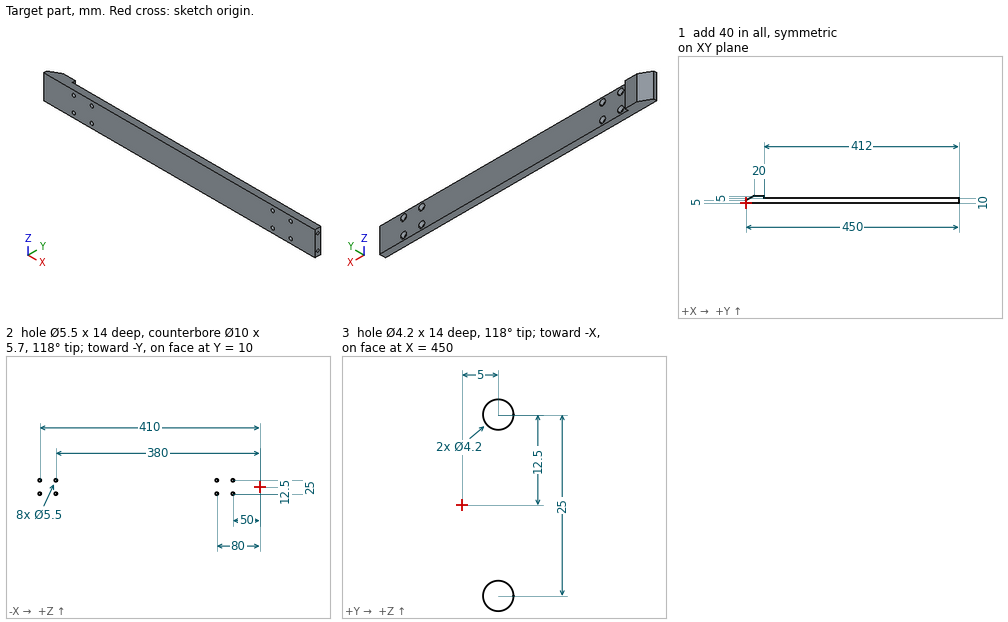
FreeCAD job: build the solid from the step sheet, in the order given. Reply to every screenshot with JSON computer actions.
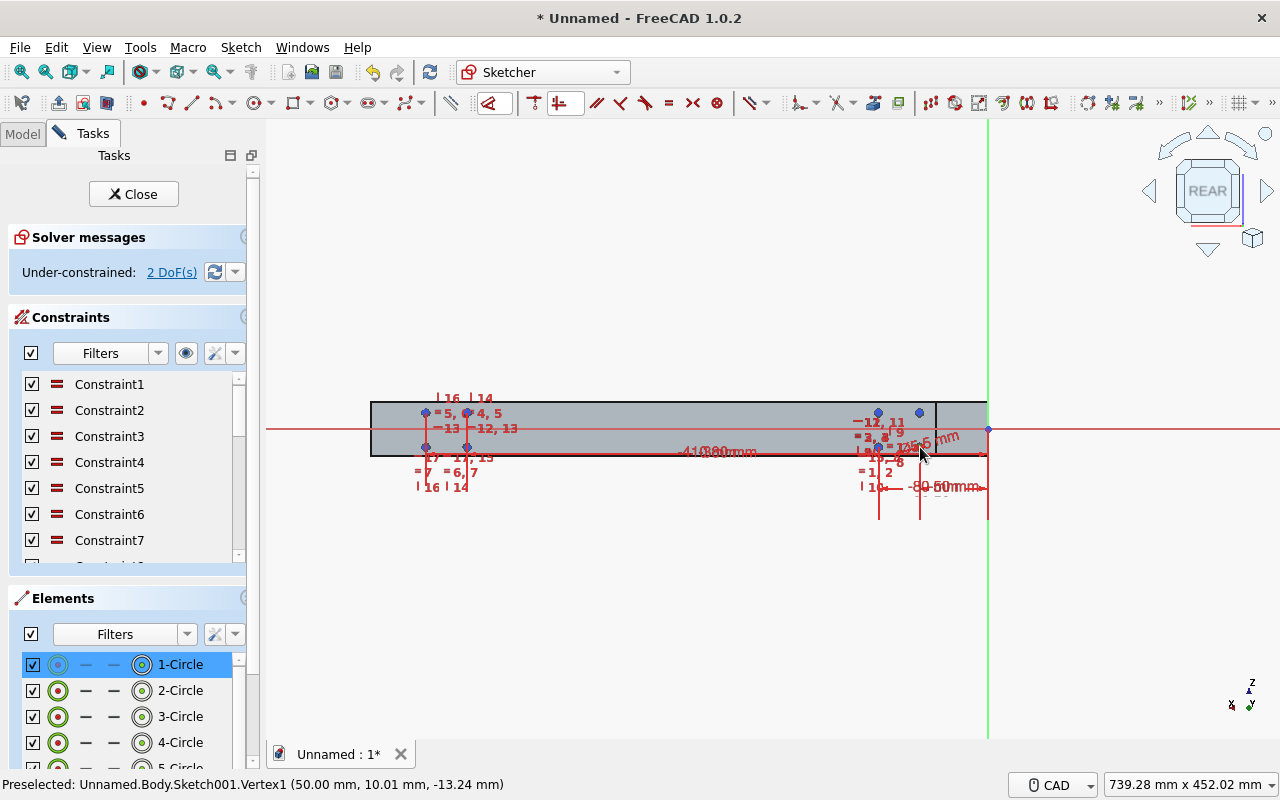
{"action": "left_click", "coordinate": [920, 413]}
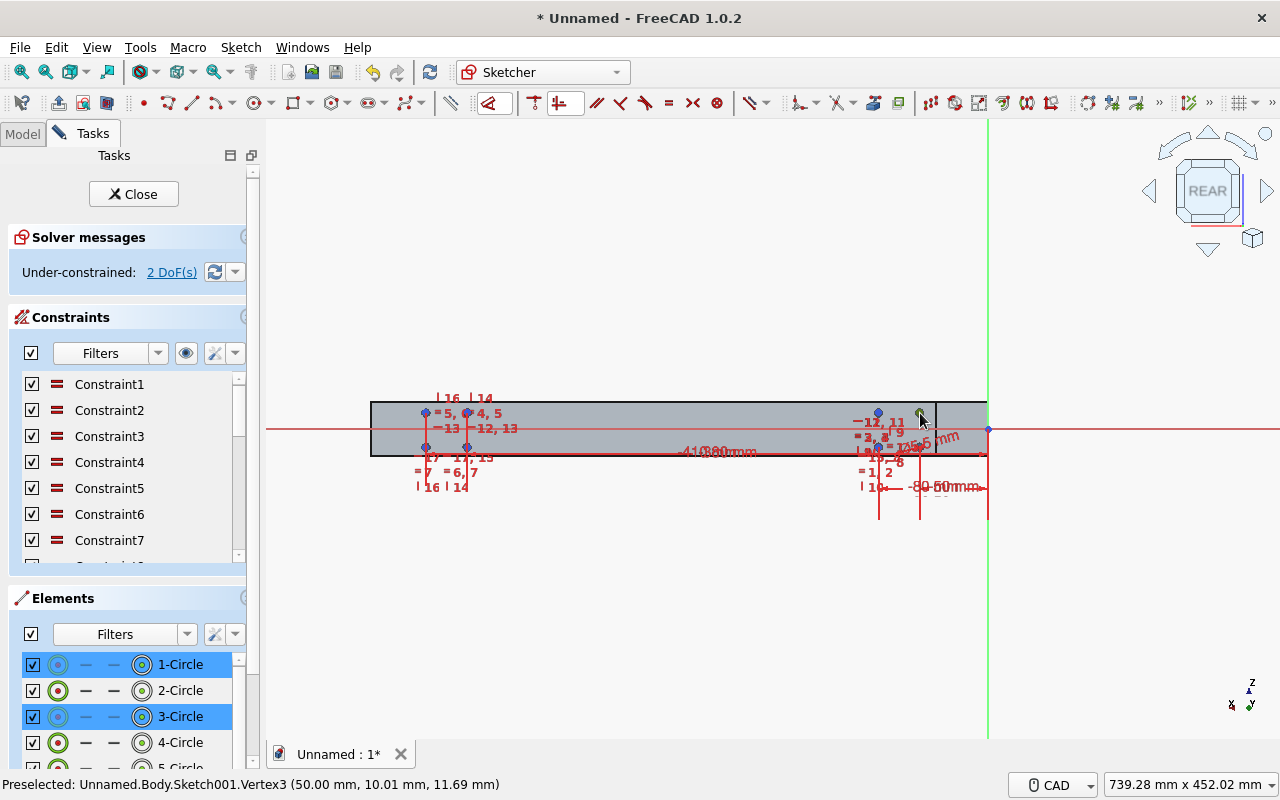
{"action": "key", "text": "i"}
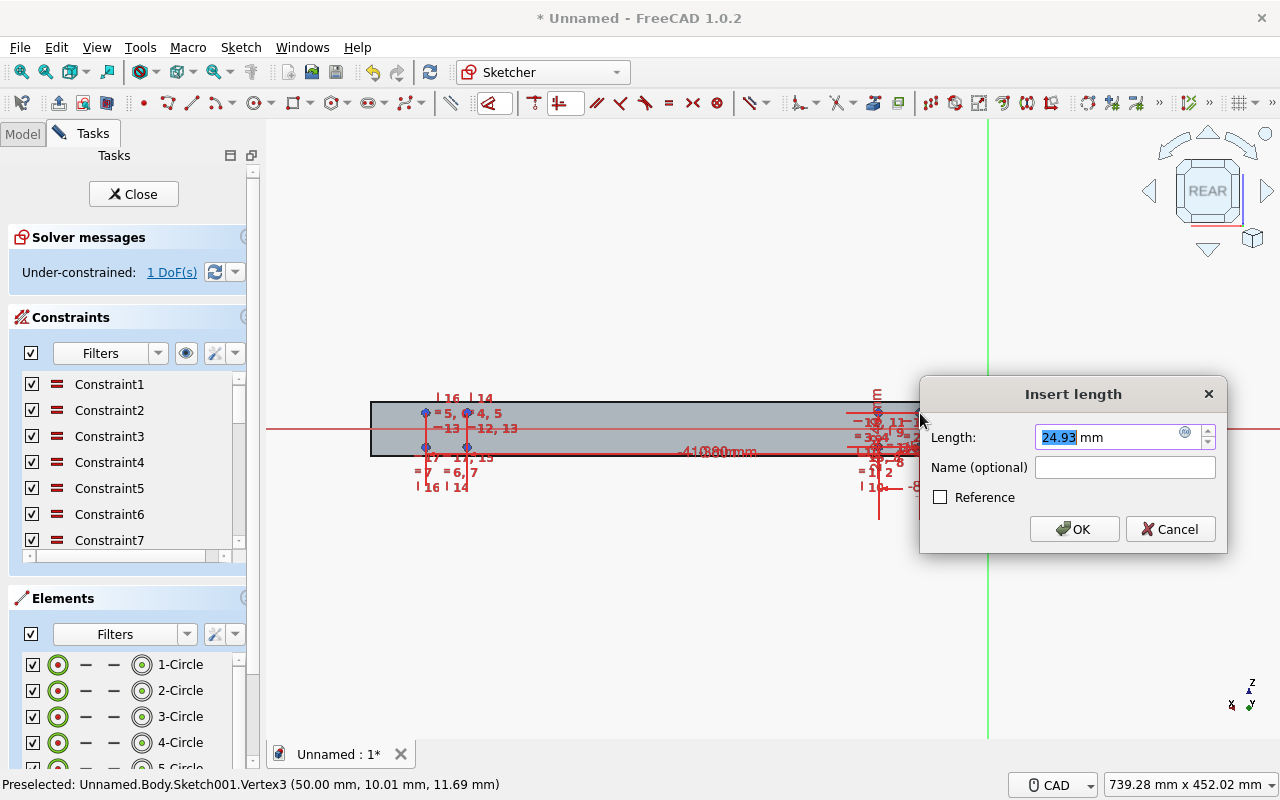
{"action": "type", "text": "25"}
{"action": "key", "text": "Return"}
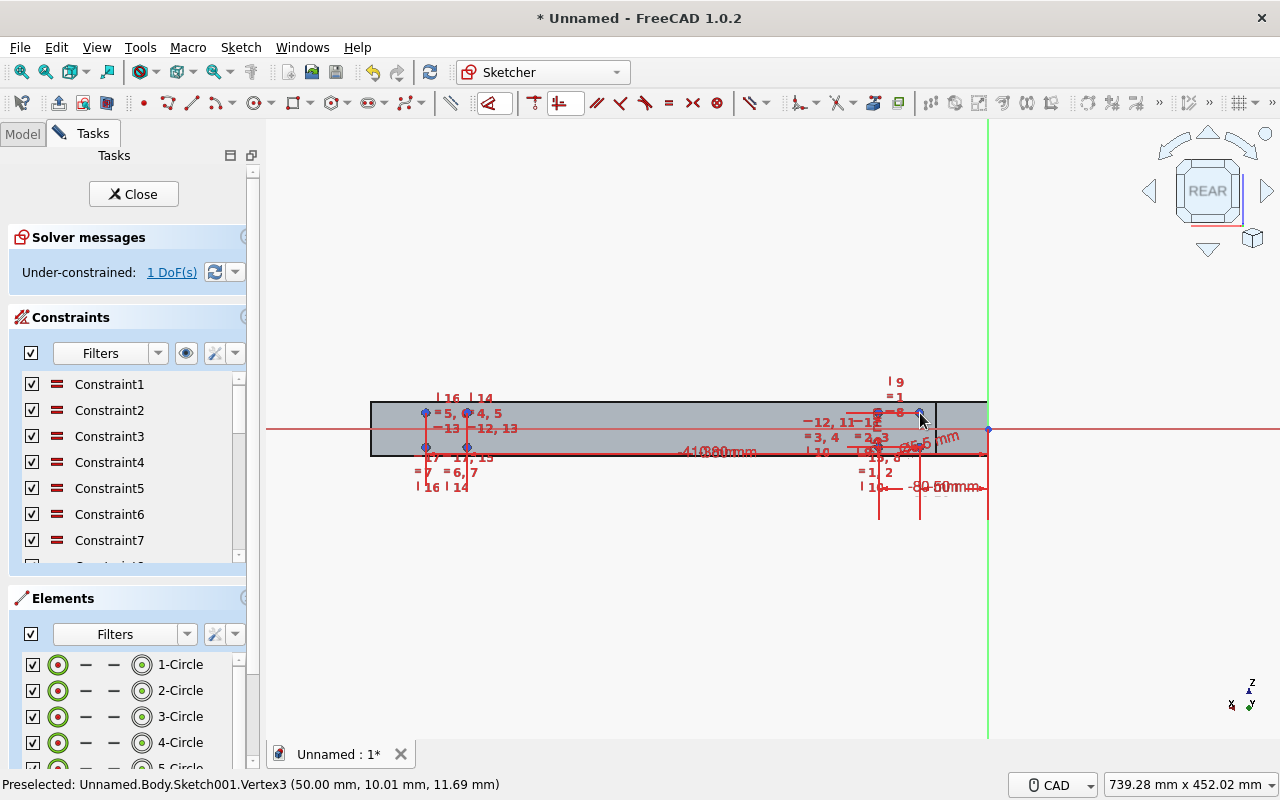
{"action": "scroll", "coordinate": [920, 447], "scroll_direction": "up", "scroll_amount": 5}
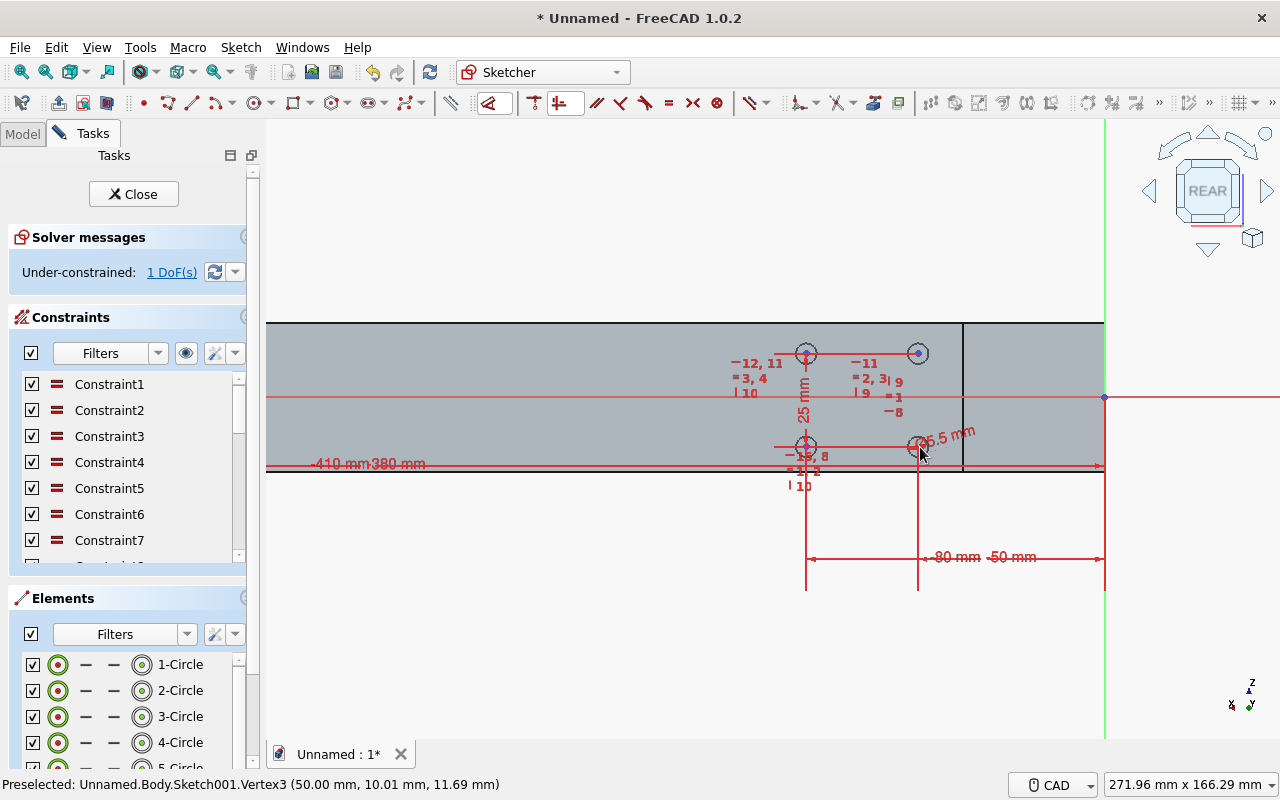
{"action": "left_click", "coordinate": [918, 447]}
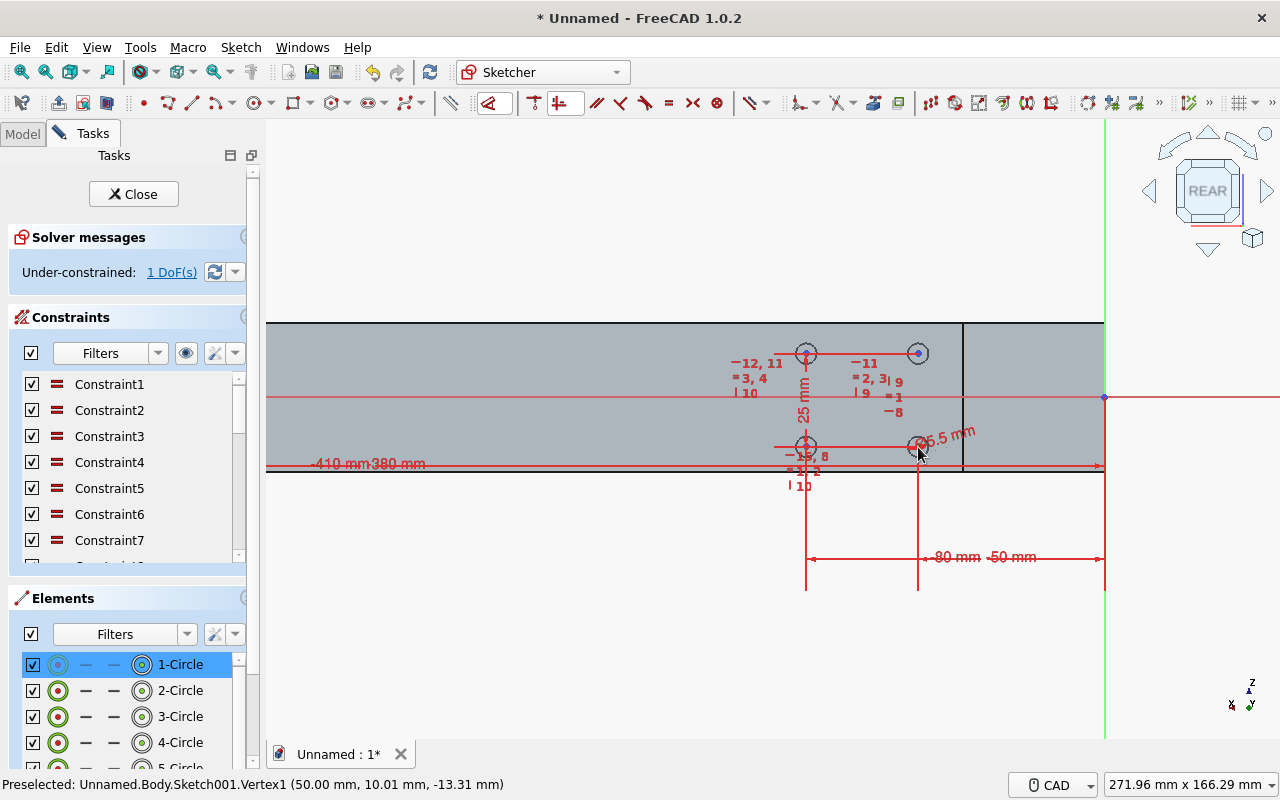
{"action": "key", "text": "i"}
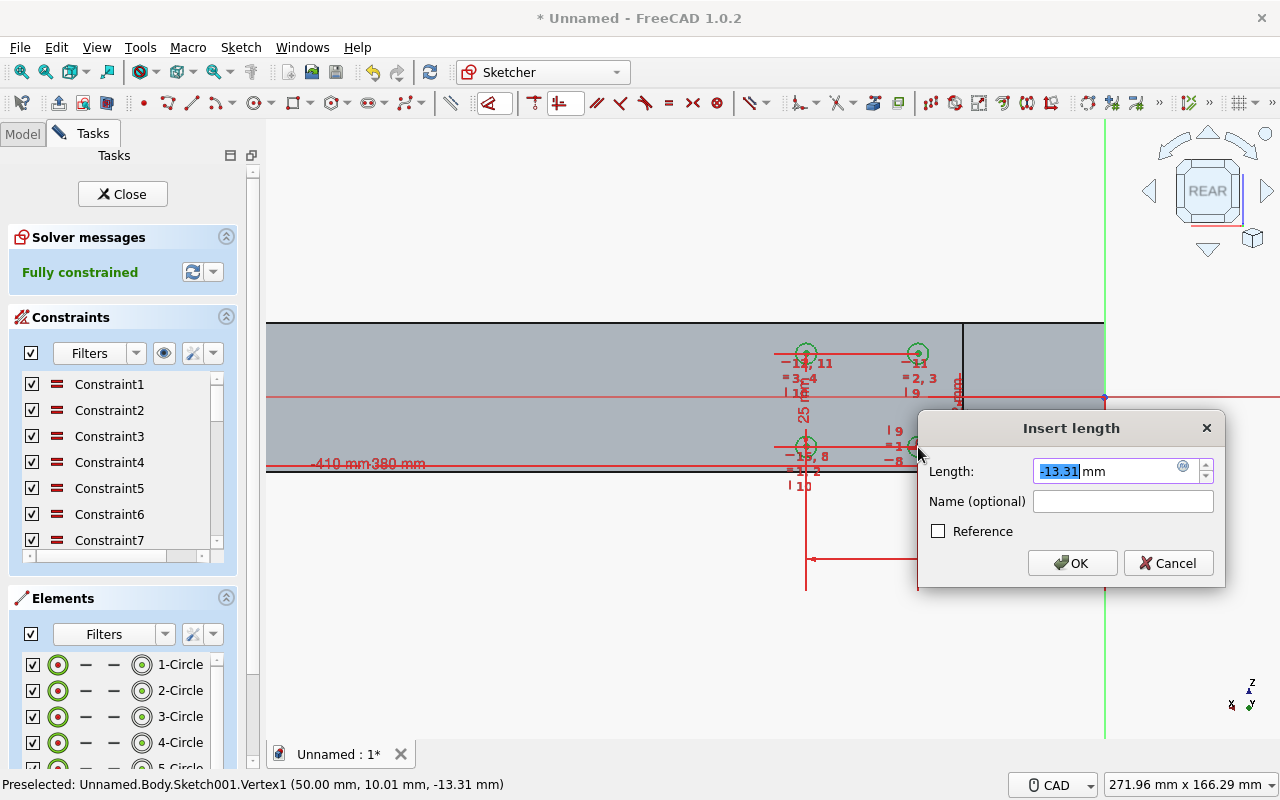
{"action": "type", "text": "-12.5"}
{"action": "key", "text": "Return"}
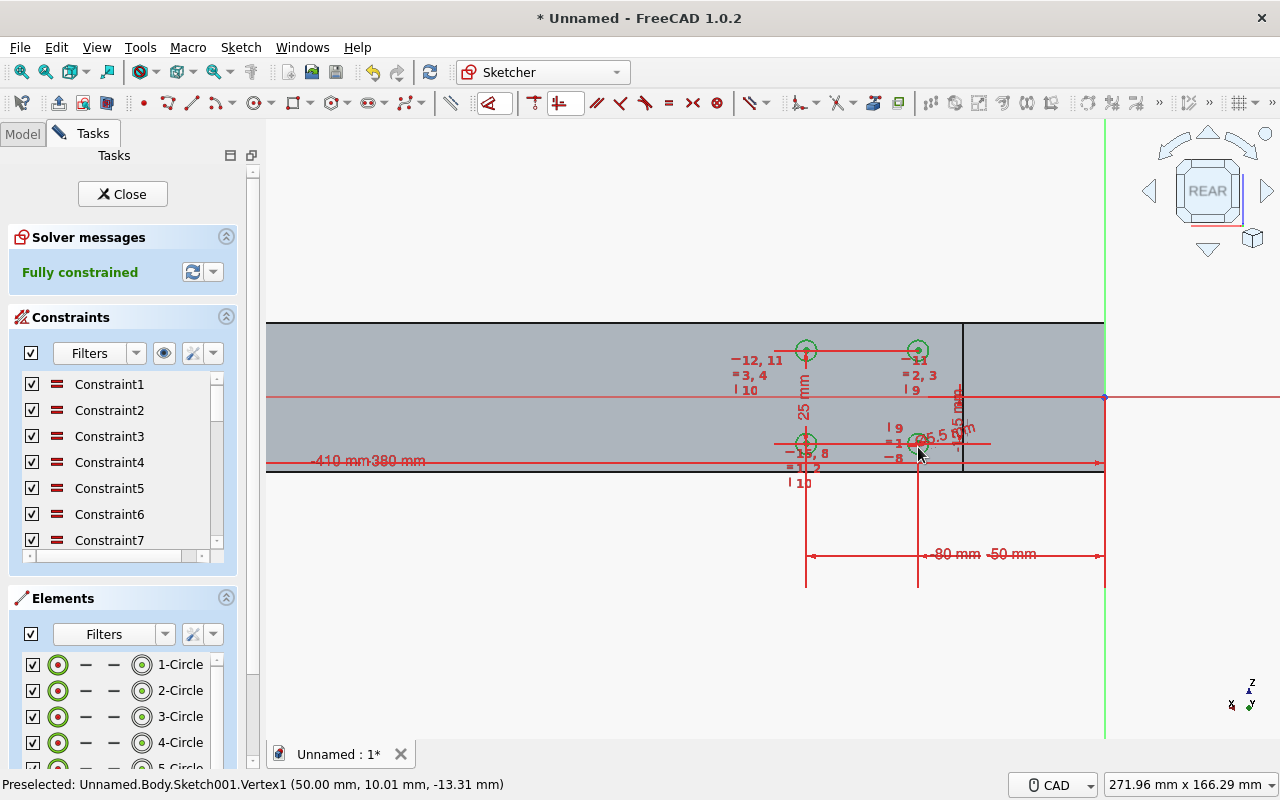
{"action": "left_click", "coordinate": [123, 194]}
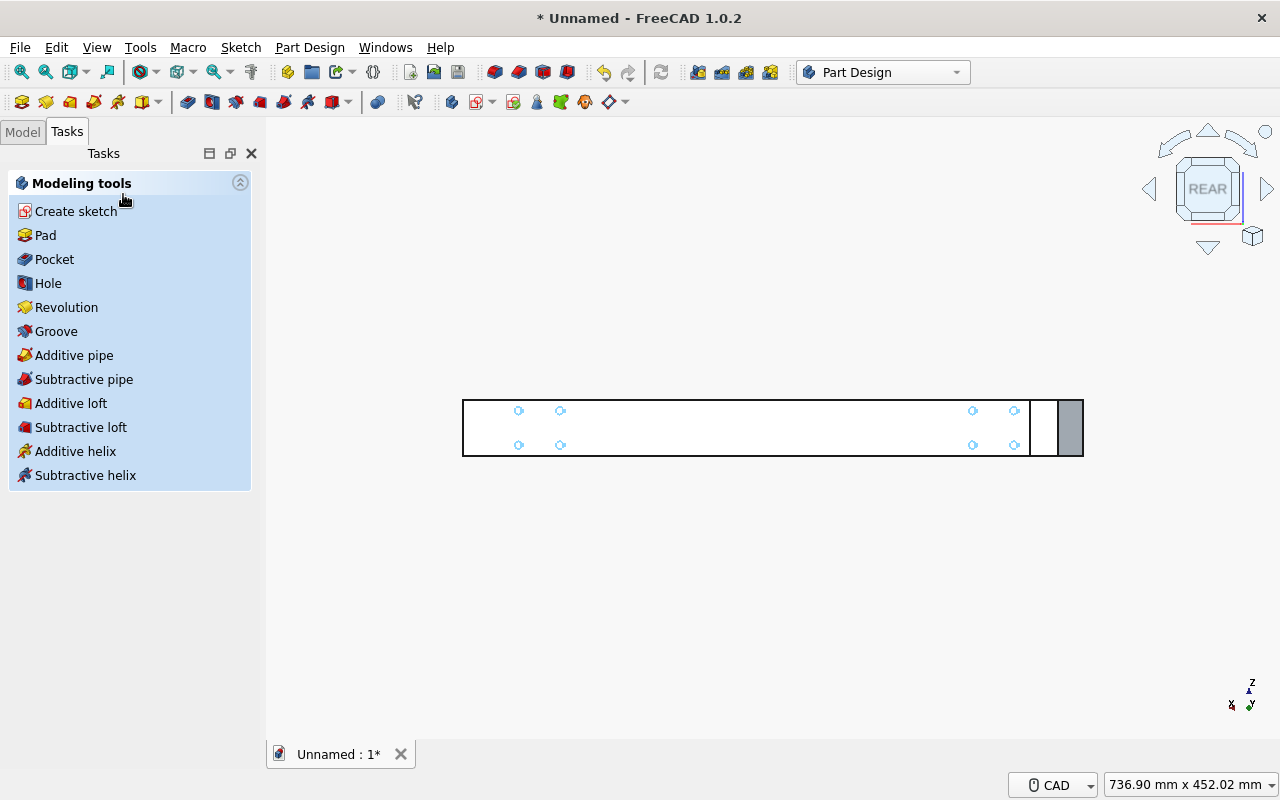
{"action": "left_click", "coordinate": [212, 102]}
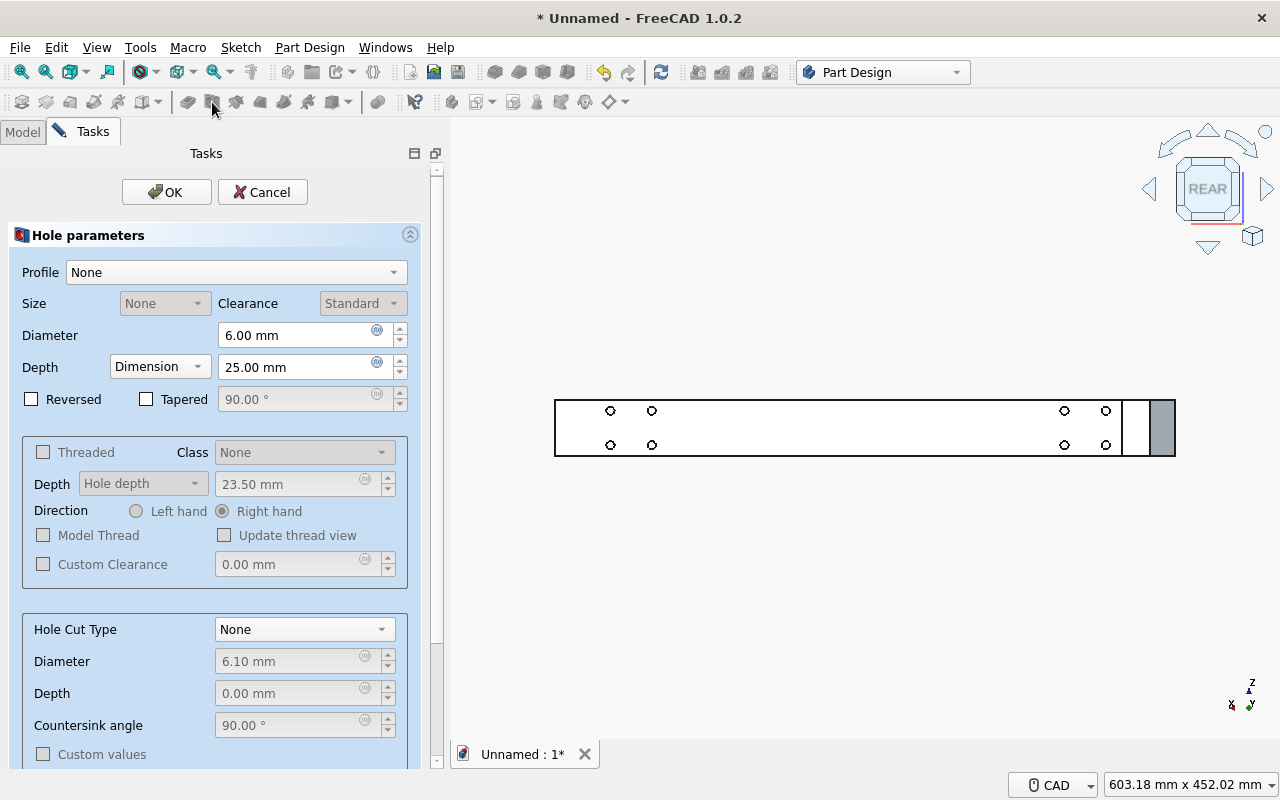
{"action": "triple_click", "coordinate": [305, 335]}